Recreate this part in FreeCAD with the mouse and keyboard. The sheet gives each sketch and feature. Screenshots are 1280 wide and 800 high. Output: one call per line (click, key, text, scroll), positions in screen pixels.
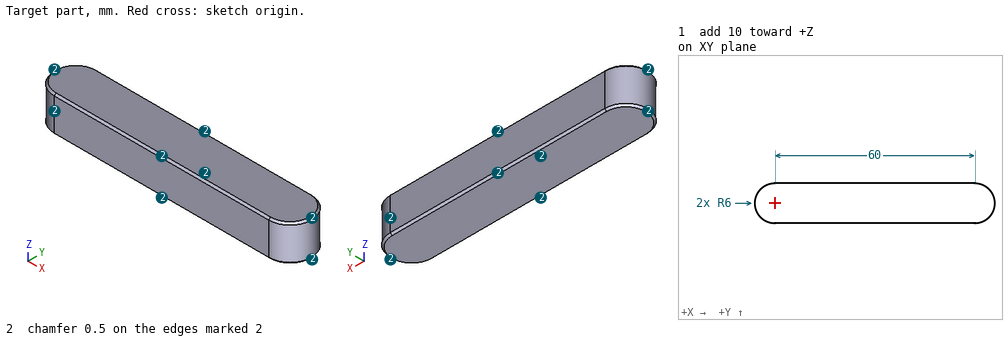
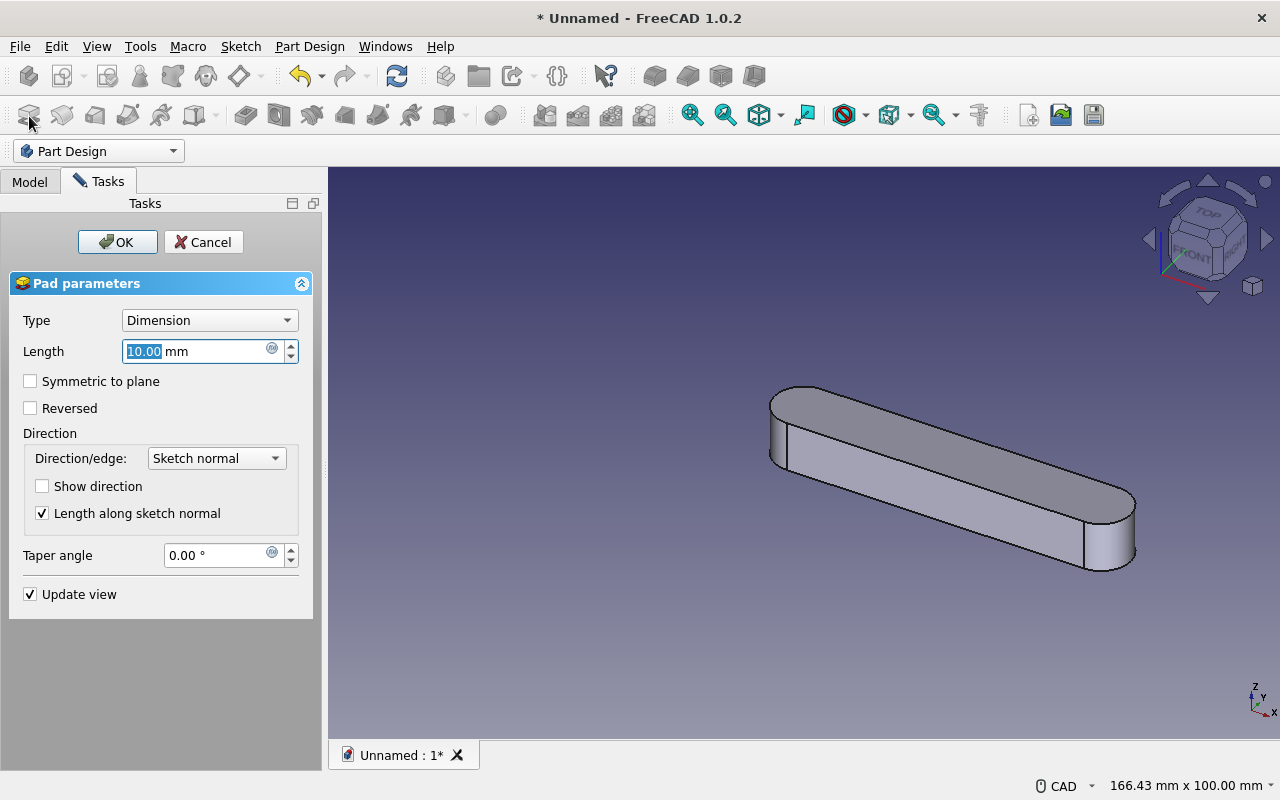
text(10)
key(Tab)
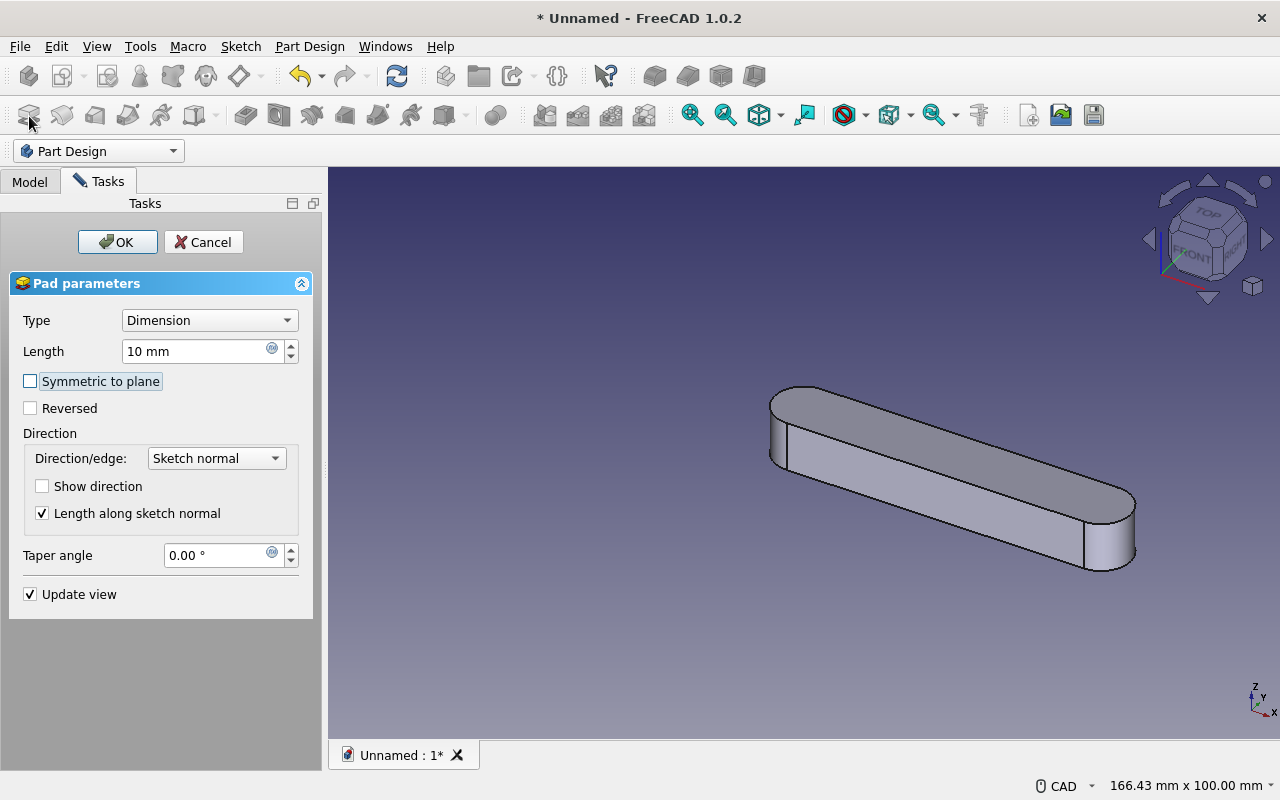
click(118, 242)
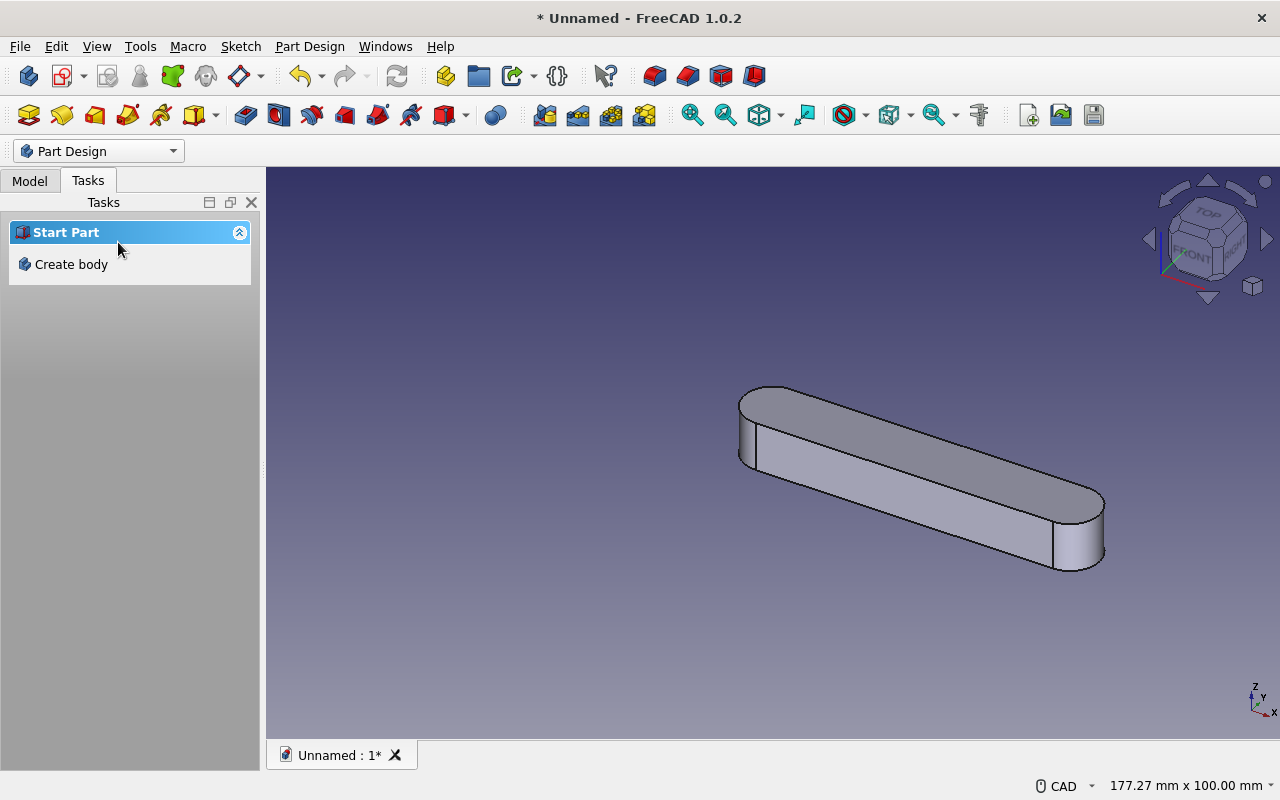
click(693, 116)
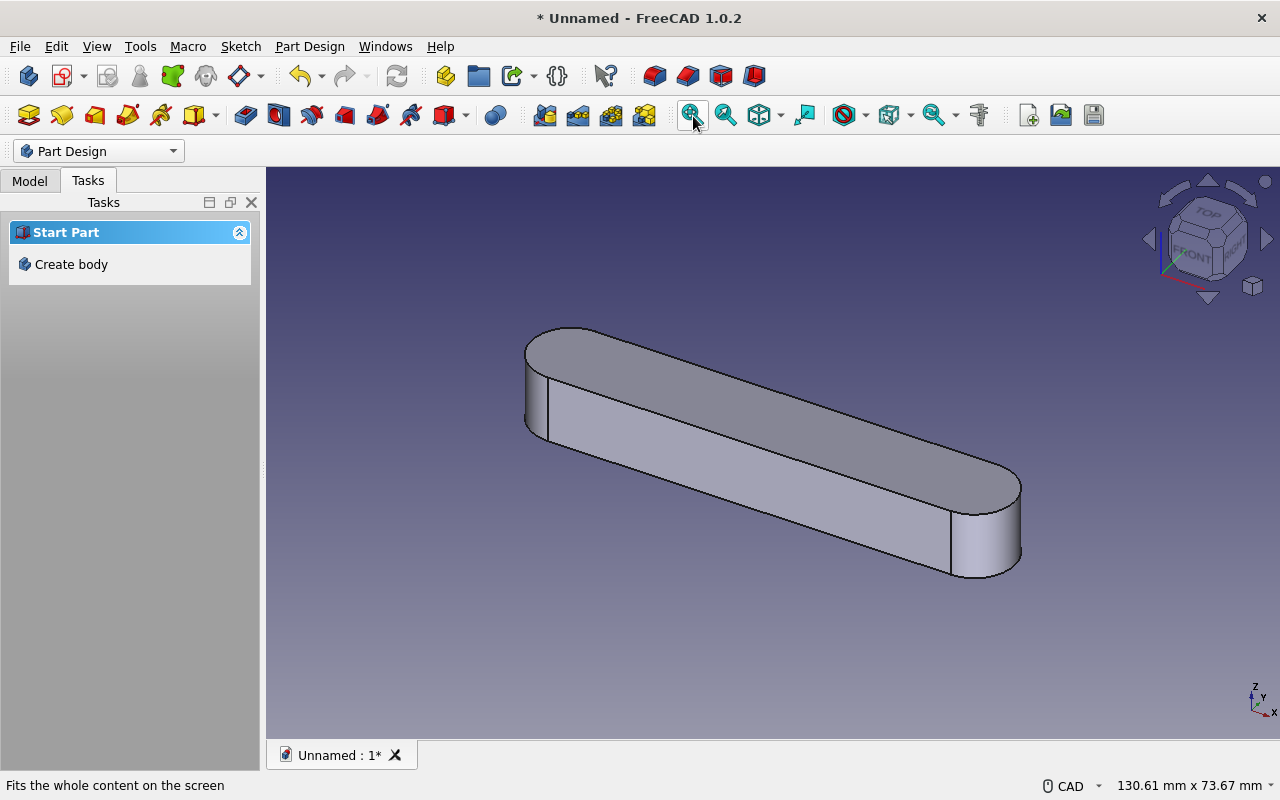
click(911, 466)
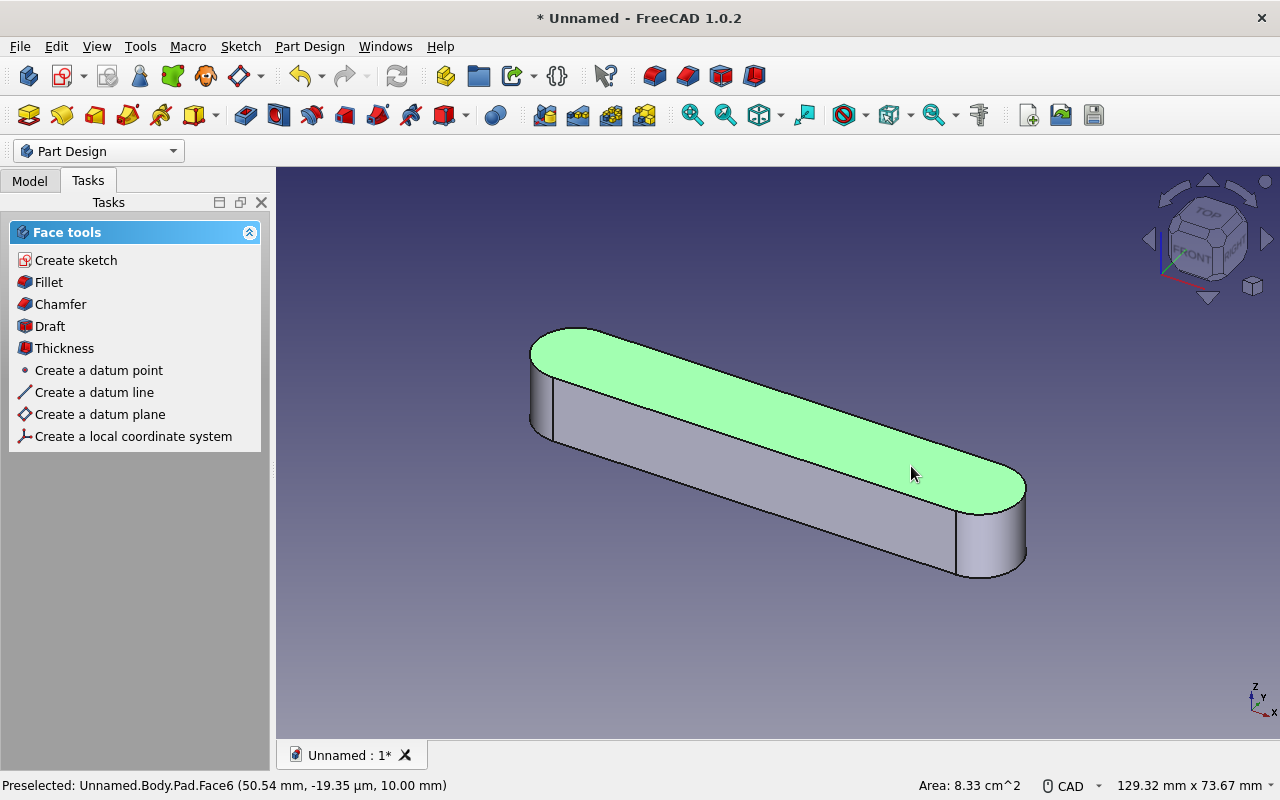
key(0)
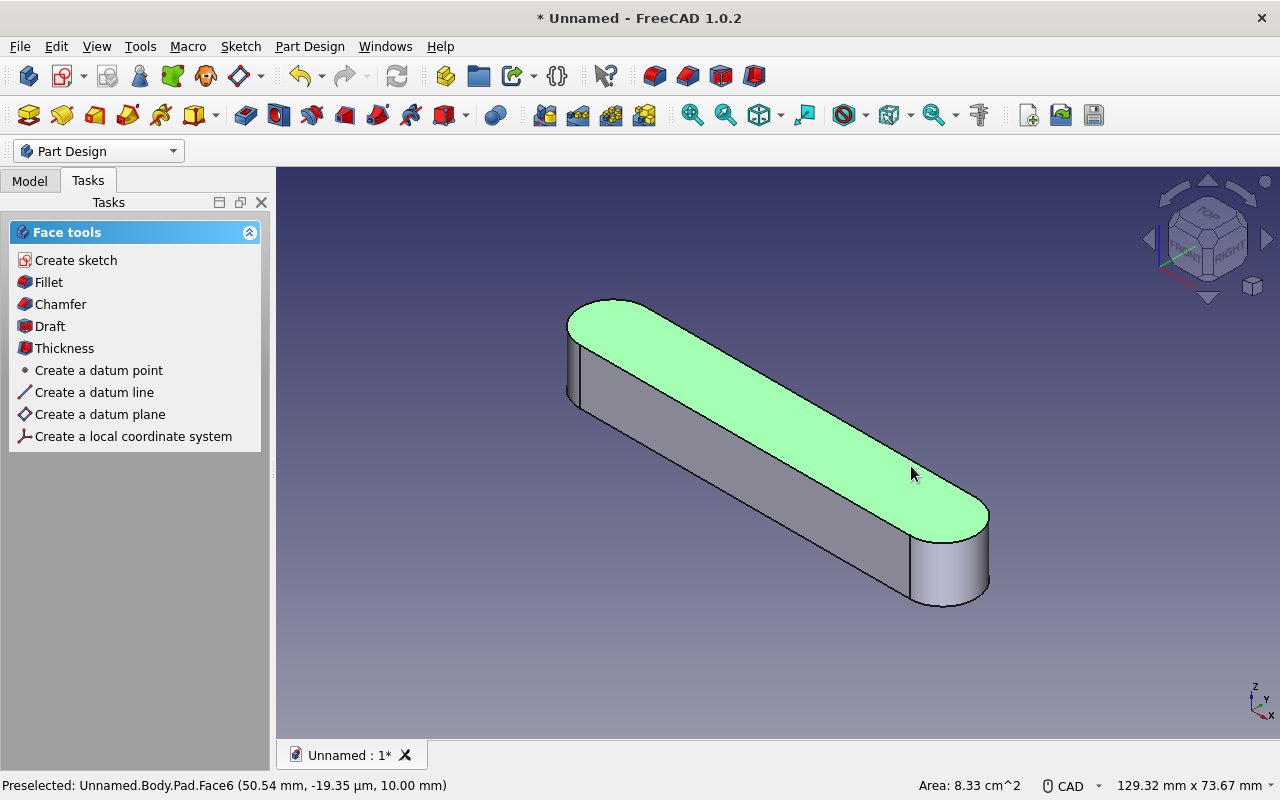
key(2)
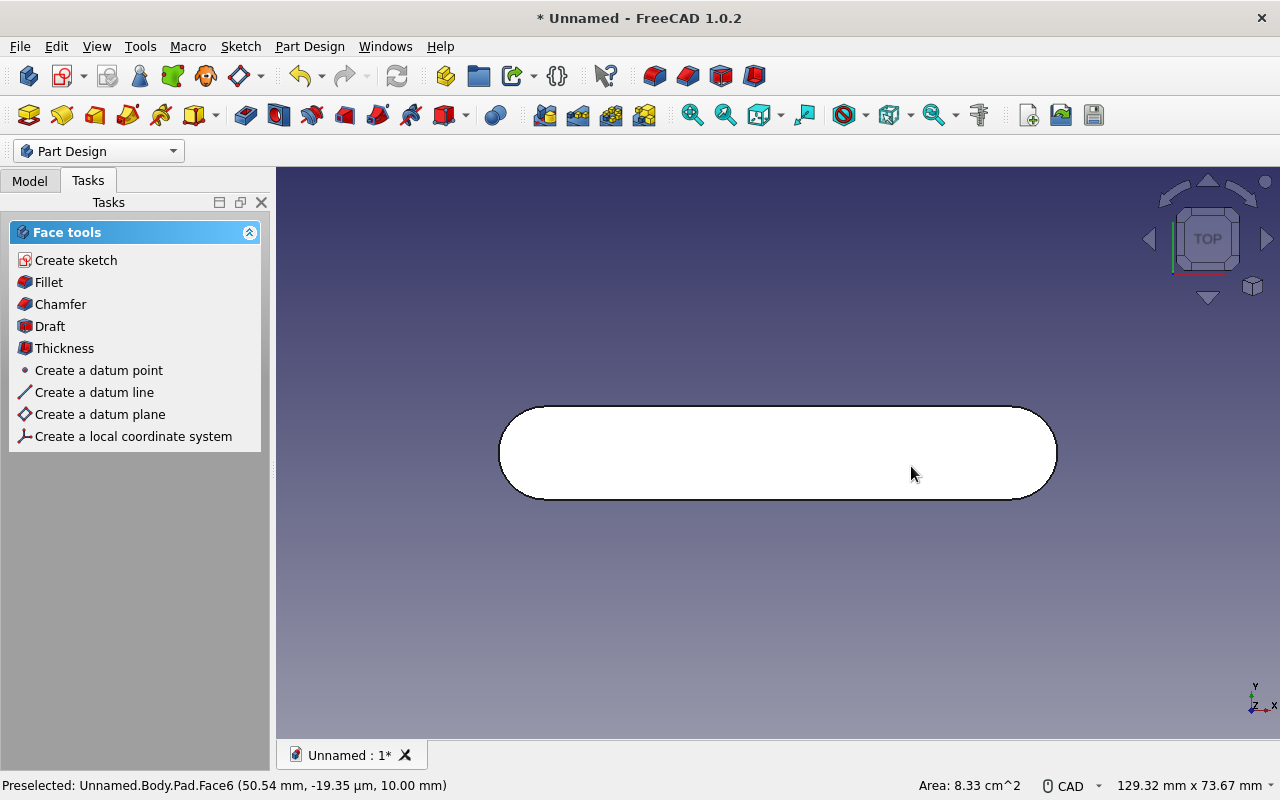
key(1)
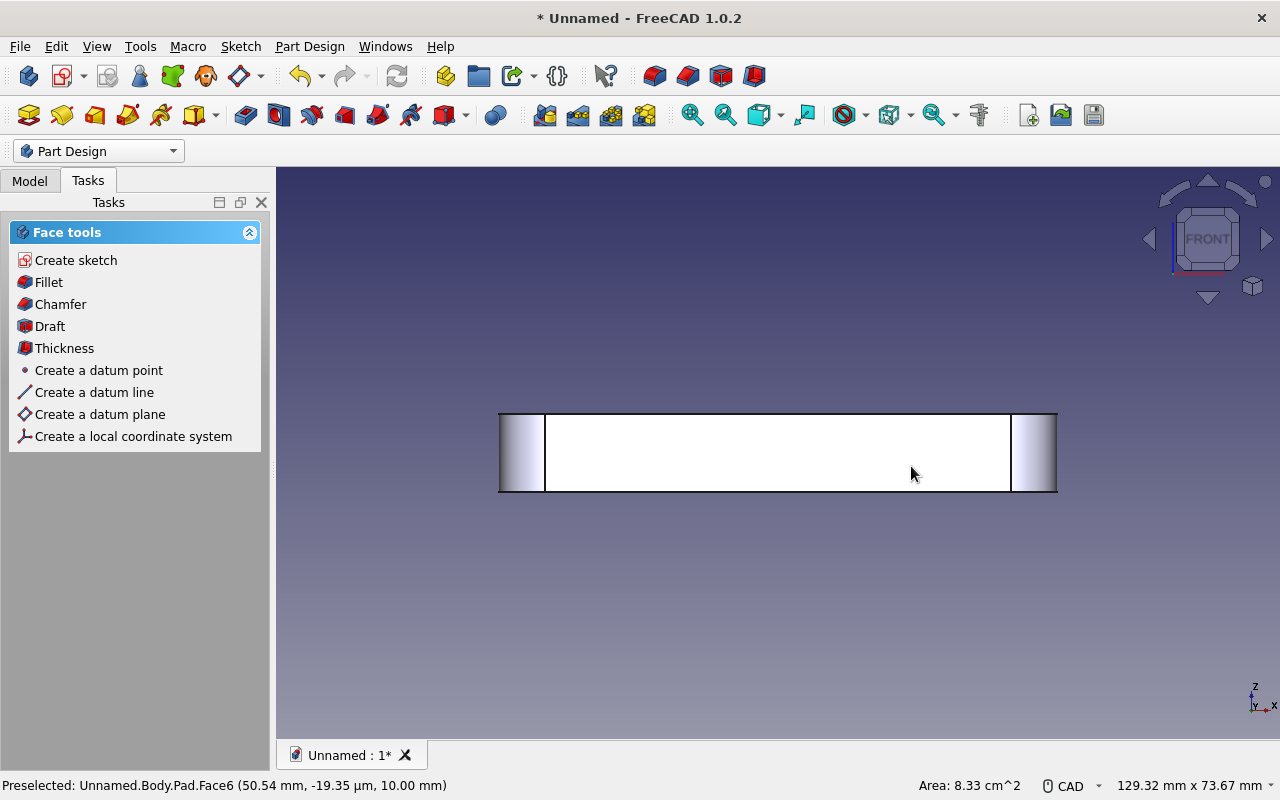
key(3)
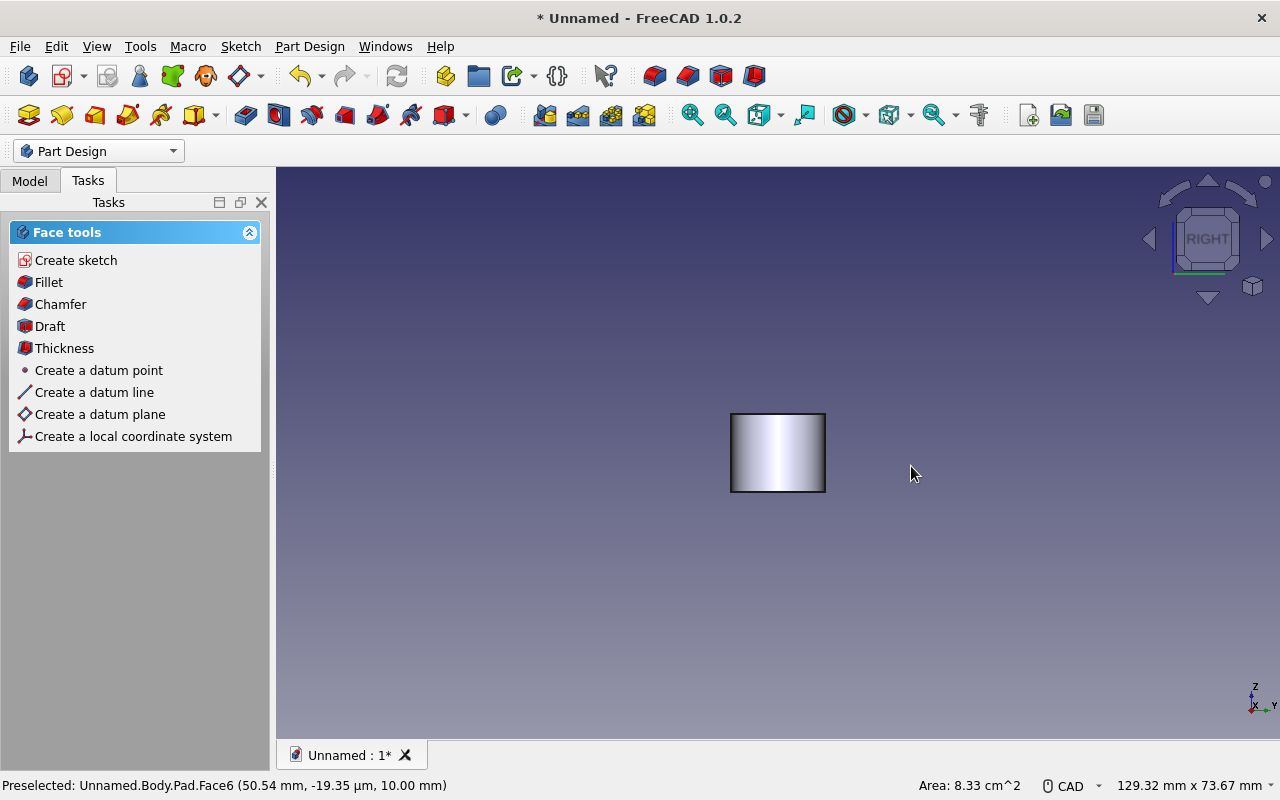
click(693, 116)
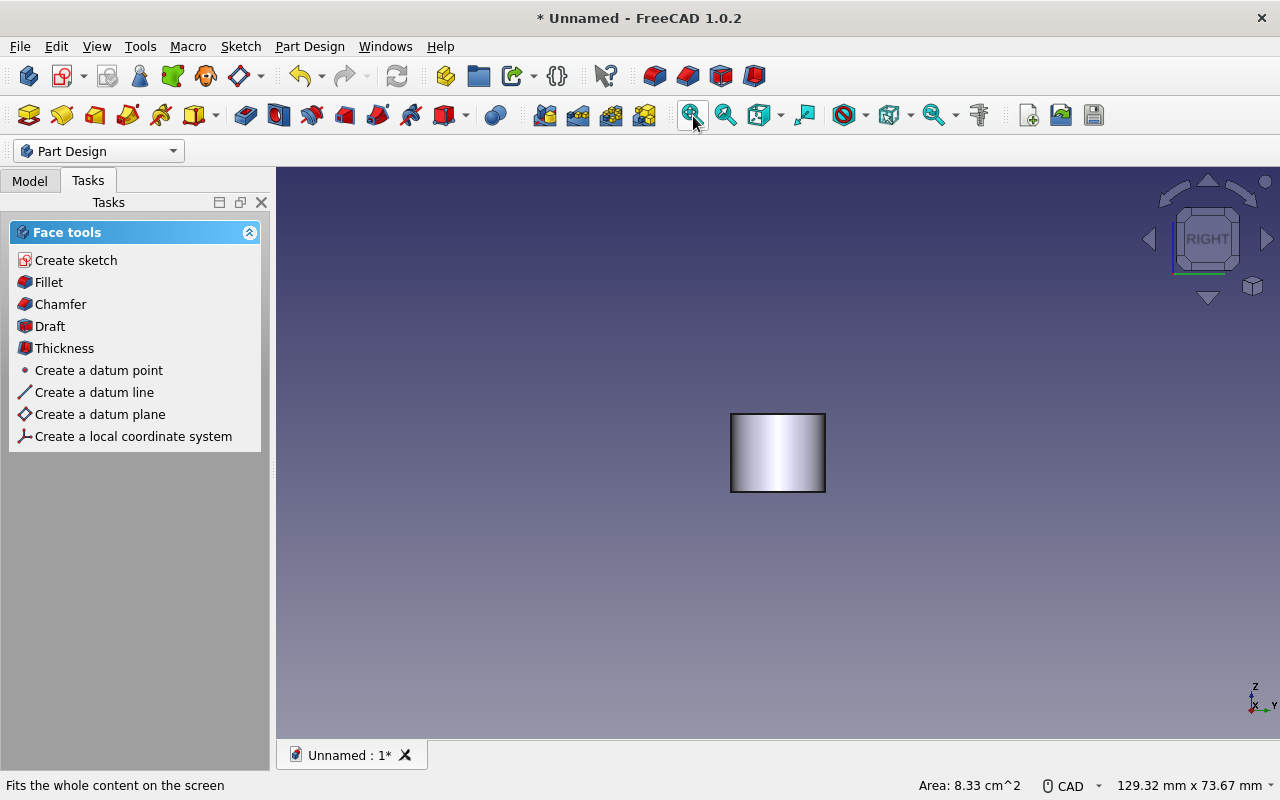
key(5)